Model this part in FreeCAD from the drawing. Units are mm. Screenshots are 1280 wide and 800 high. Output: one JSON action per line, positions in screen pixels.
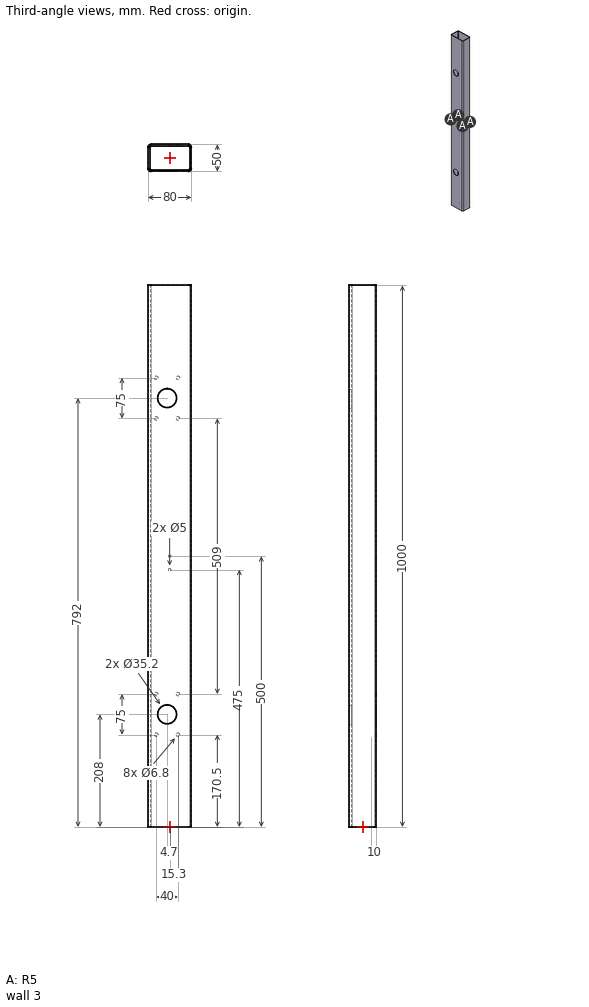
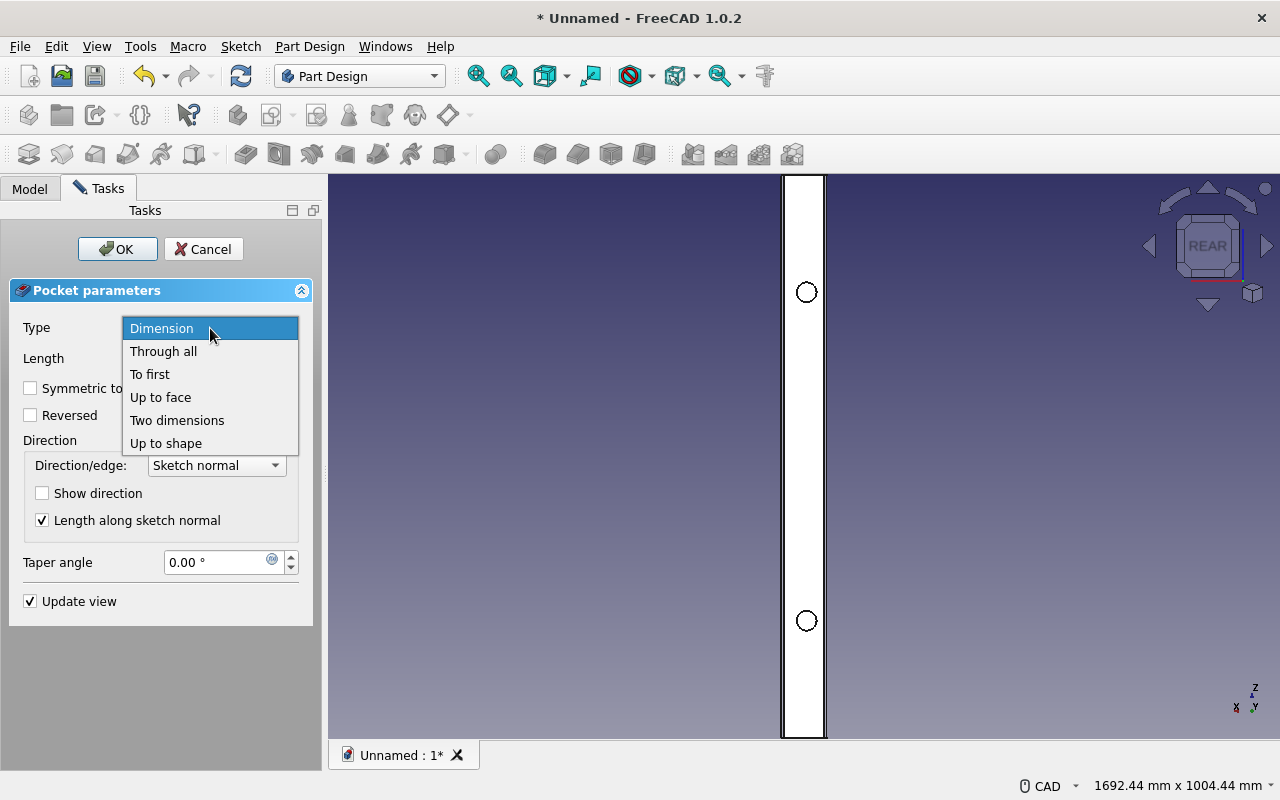
{"action": "left_click", "coordinate": [208, 352]}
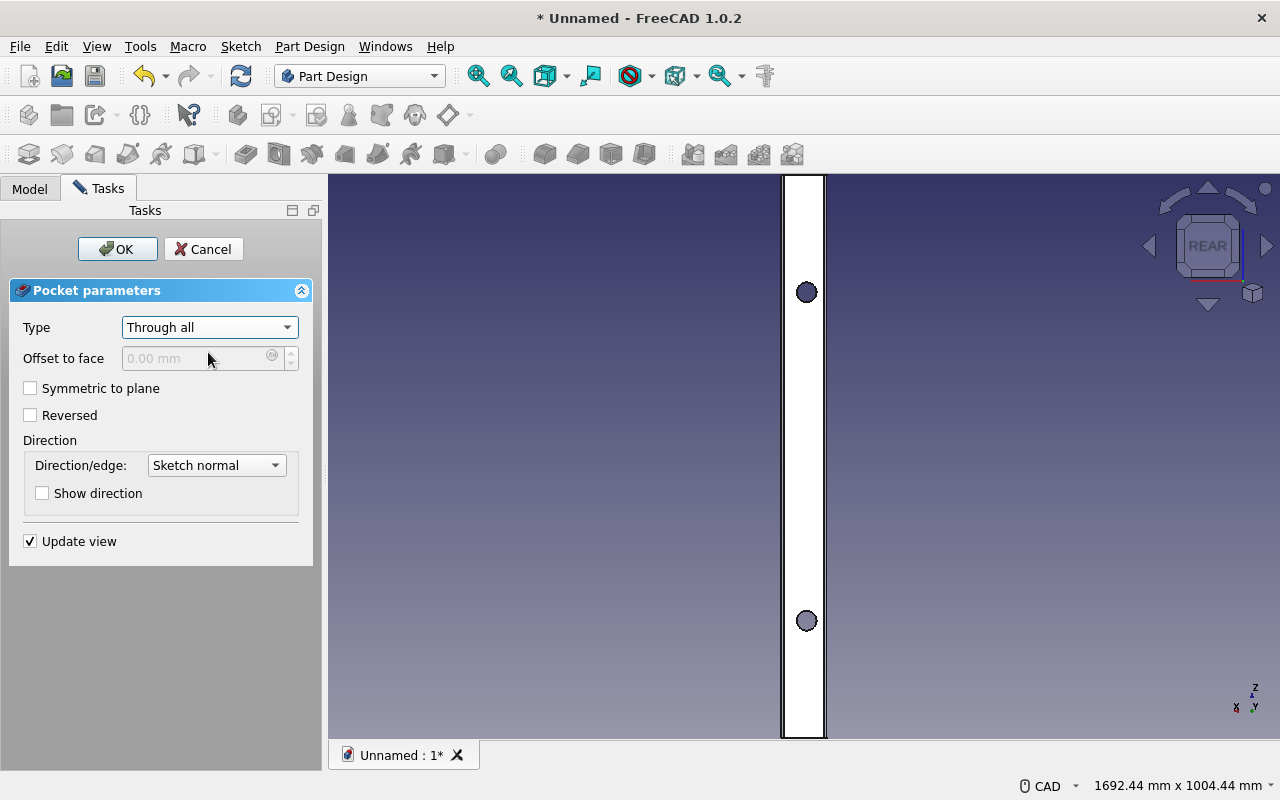
{"action": "left_click", "coordinate": [118, 249]}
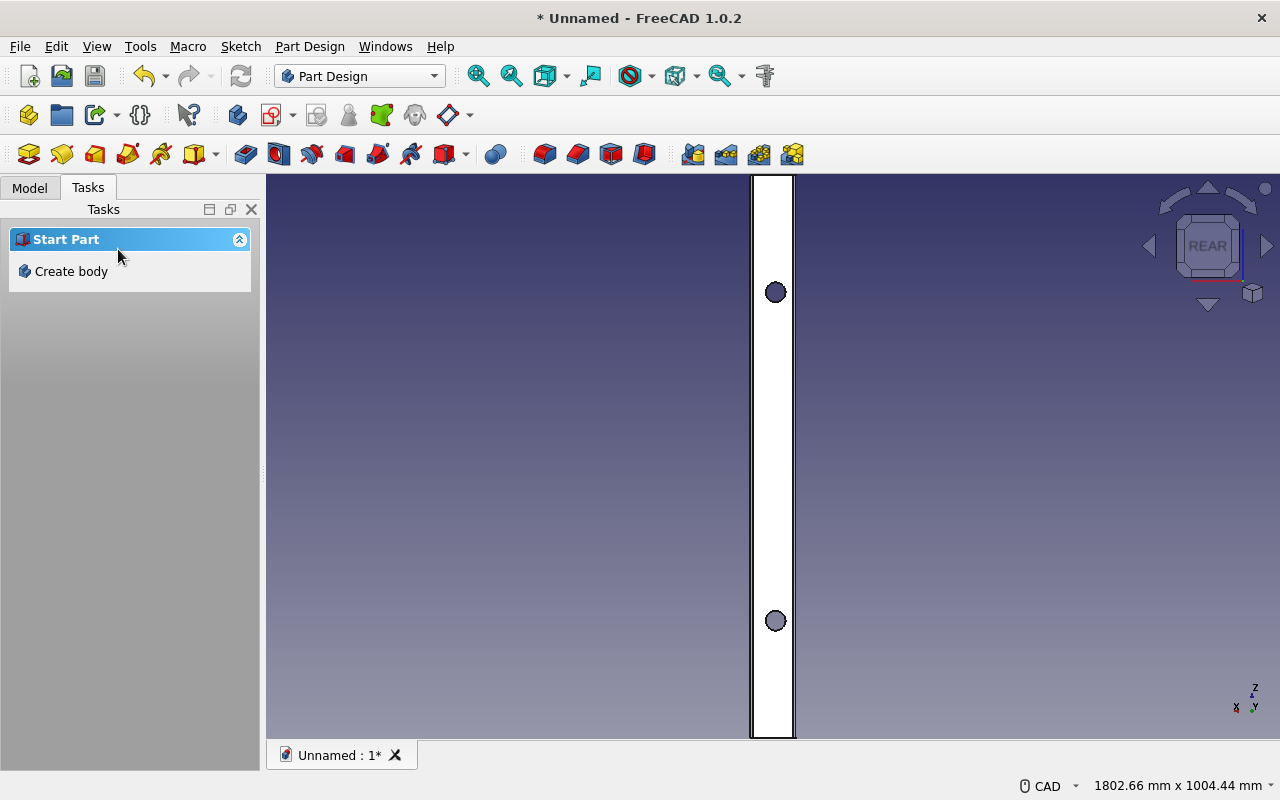
{"action": "left_click", "coordinate": [773, 214]}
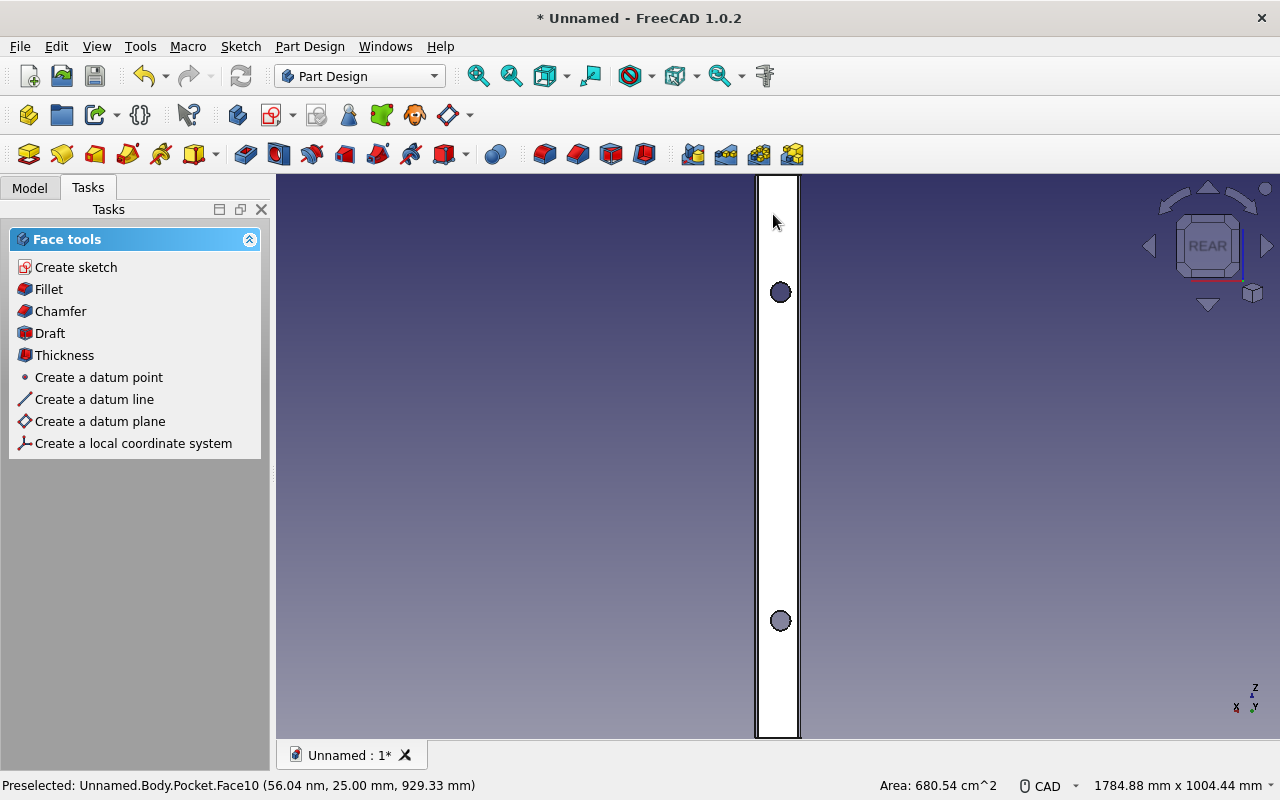
{"action": "left_click", "coordinate": [270, 116]}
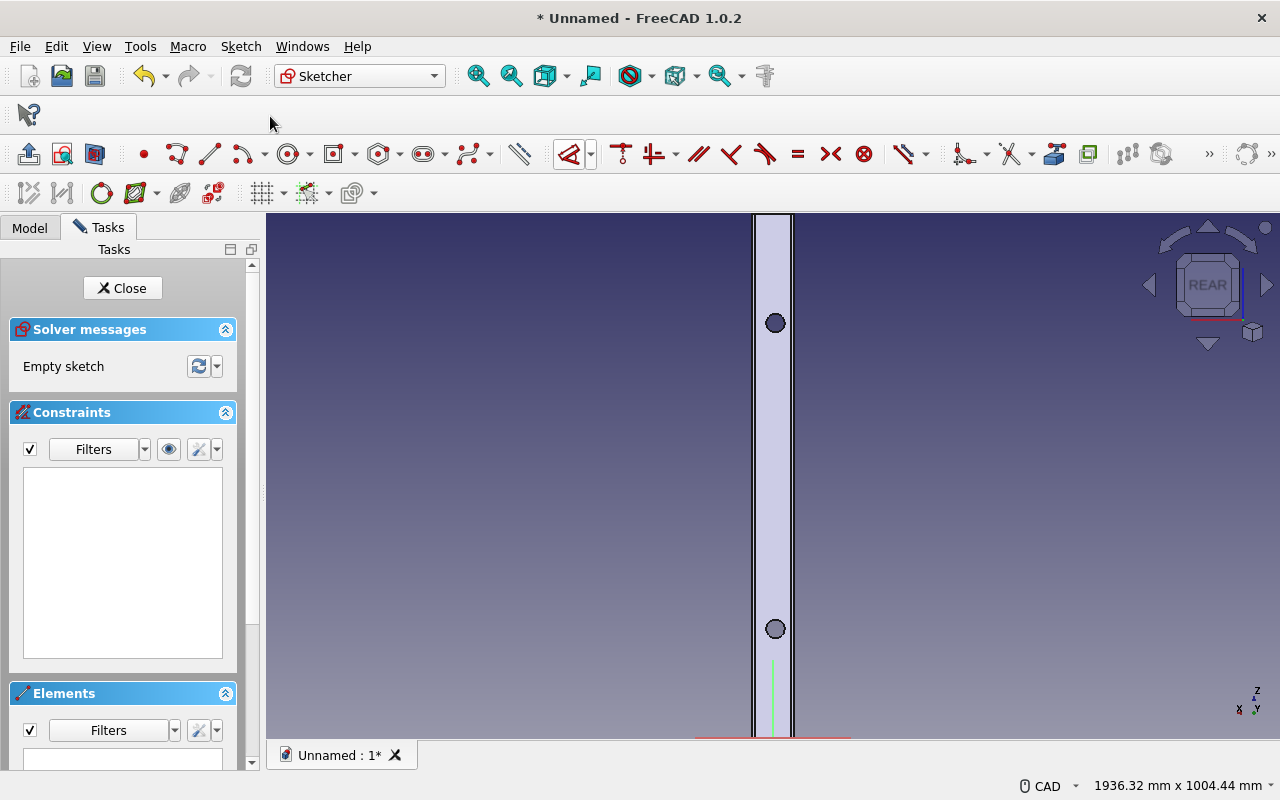
{"action": "scroll", "coordinate": [384, 278], "scroll_direction": "down", "scroll_amount": 1}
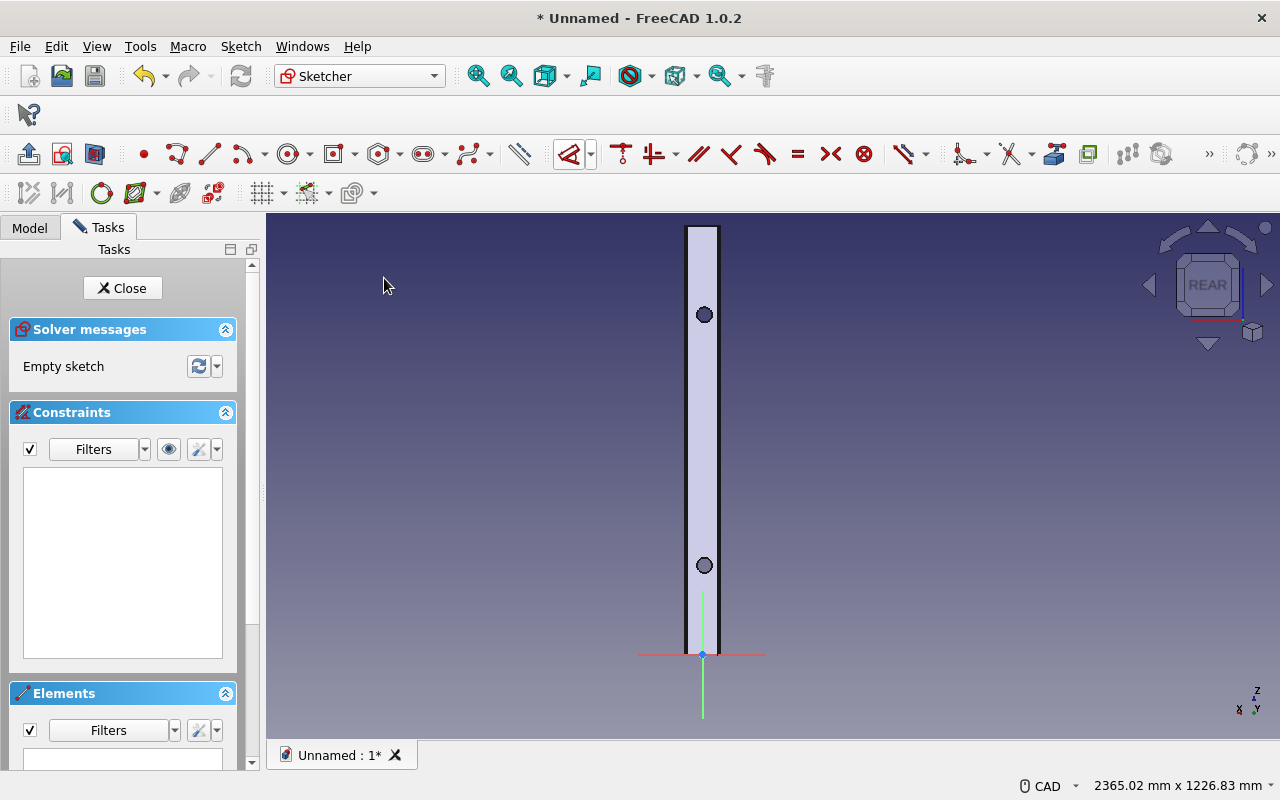
{"action": "left_click", "coordinate": [288, 154]}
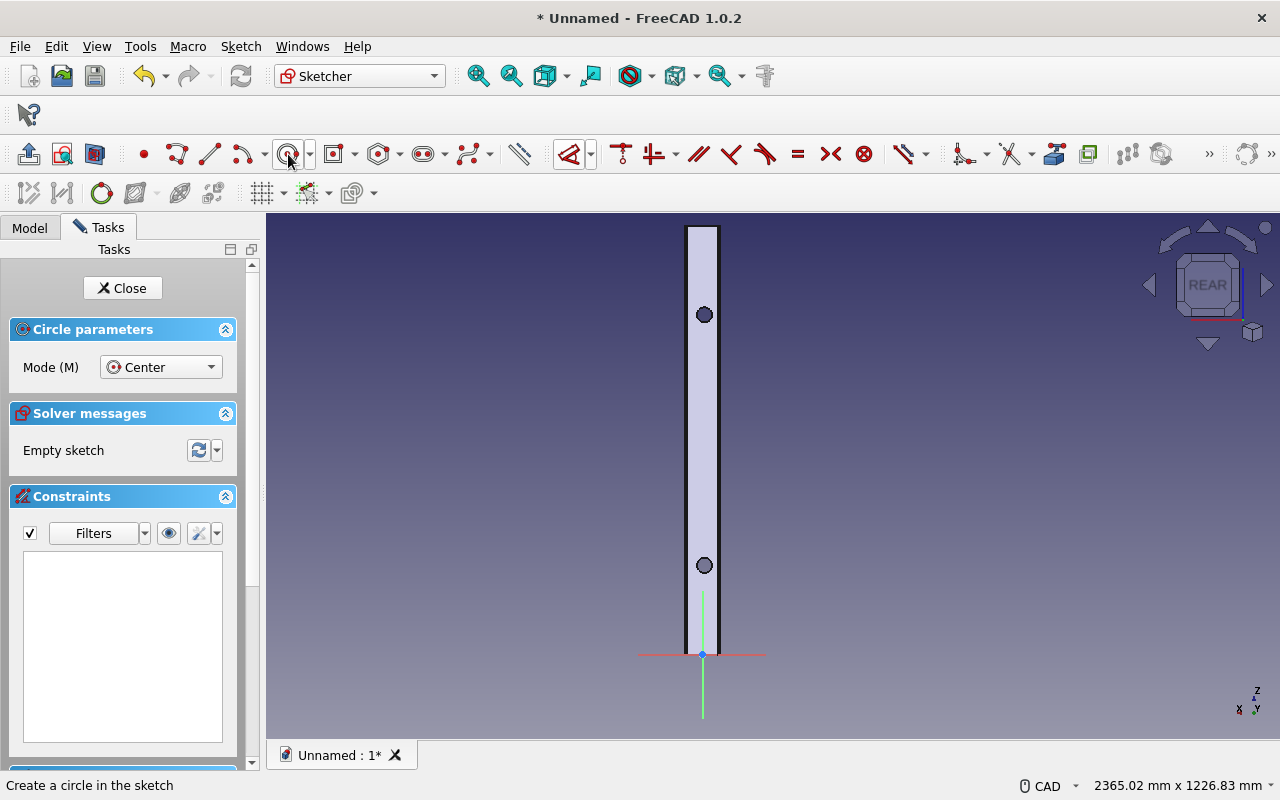
{"action": "scroll", "coordinate": [696, 581], "scroll_direction": "up", "scroll_amount": 14}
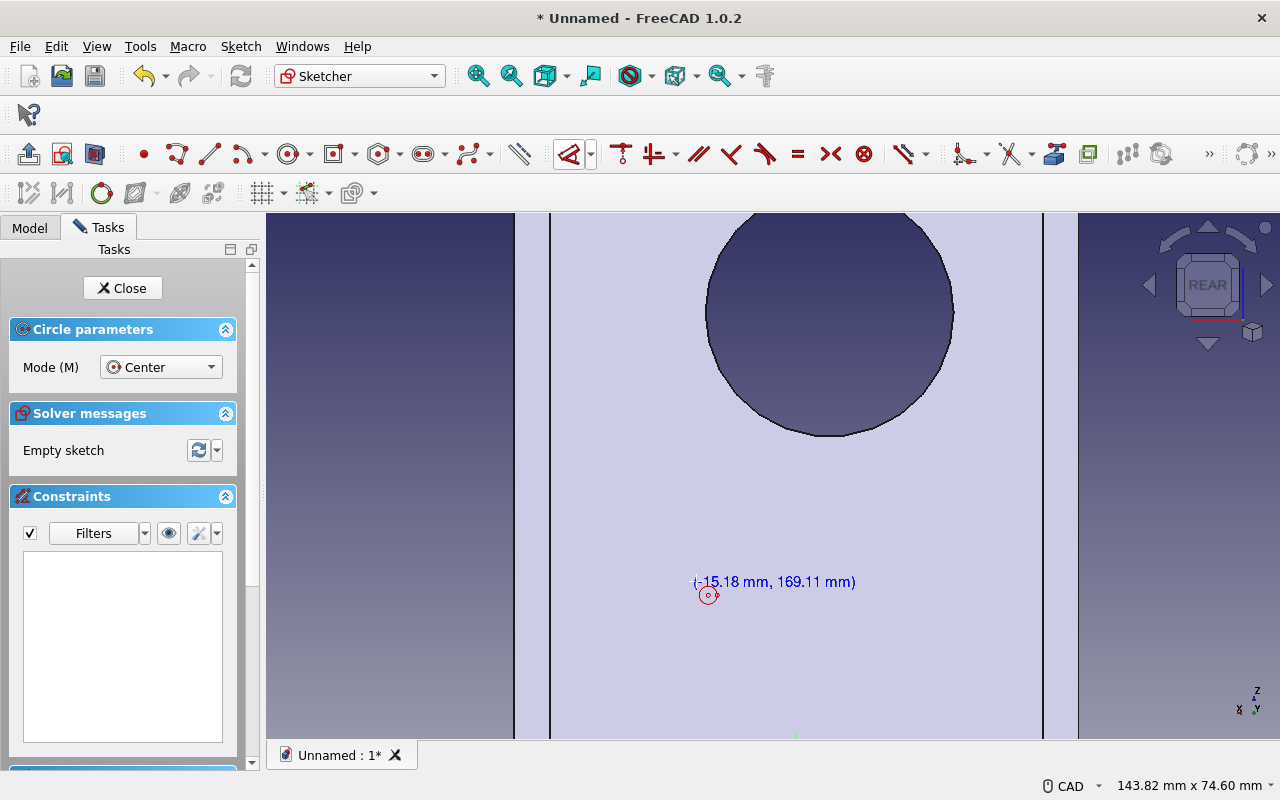
{"action": "scroll", "coordinate": [696, 582], "scroll_direction": "down", "scroll_amount": 14}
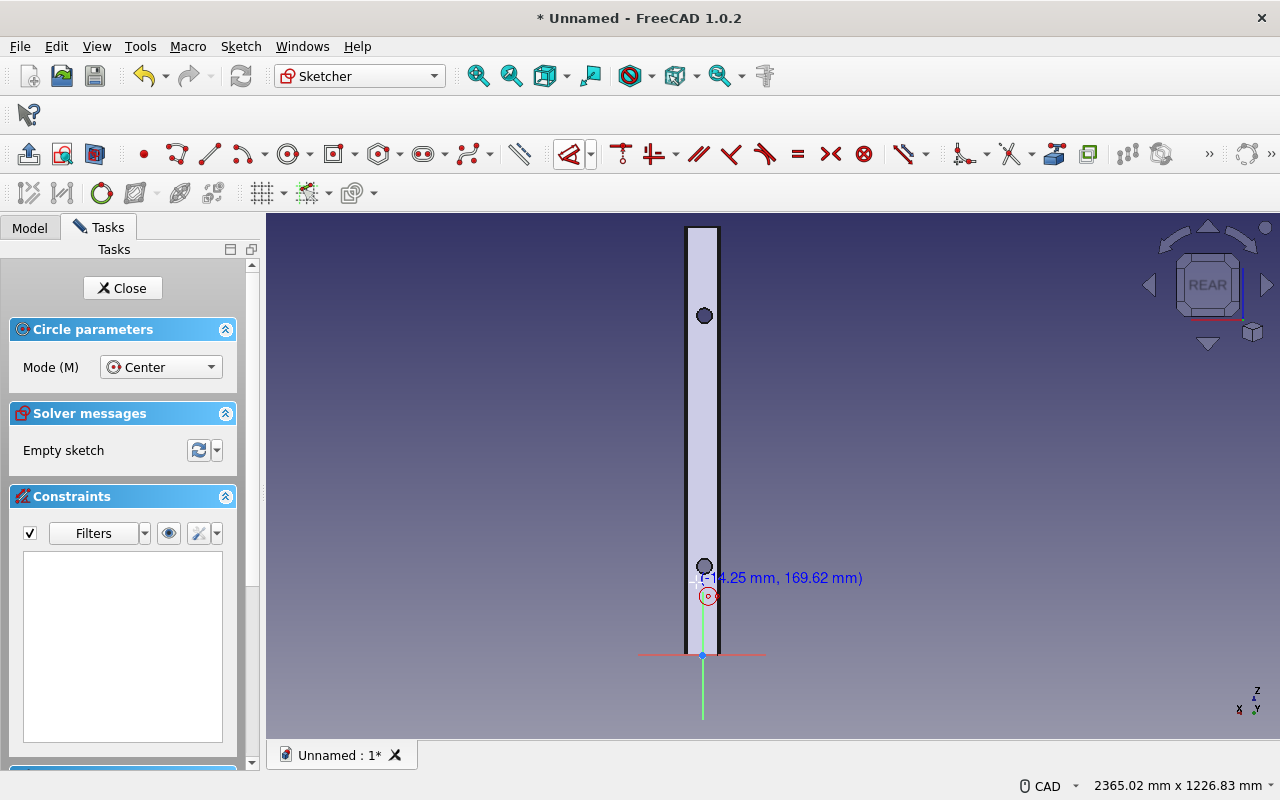
{"action": "scroll", "coordinate": [696, 582], "scroll_direction": "up", "scroll_amount": 5}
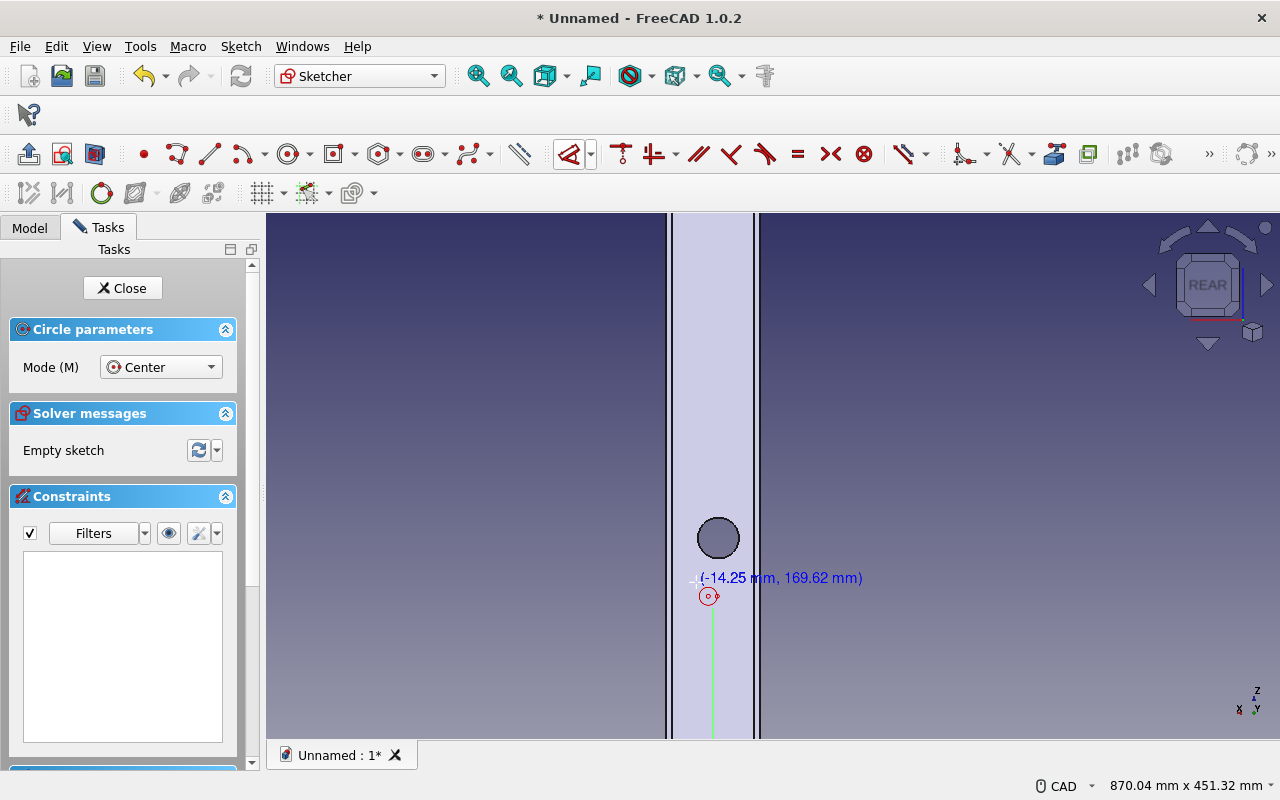
{"action": "left_click", "coordinate": [695, 582]}
{"action": "mouse_move", "coordinate": [698, 579]}